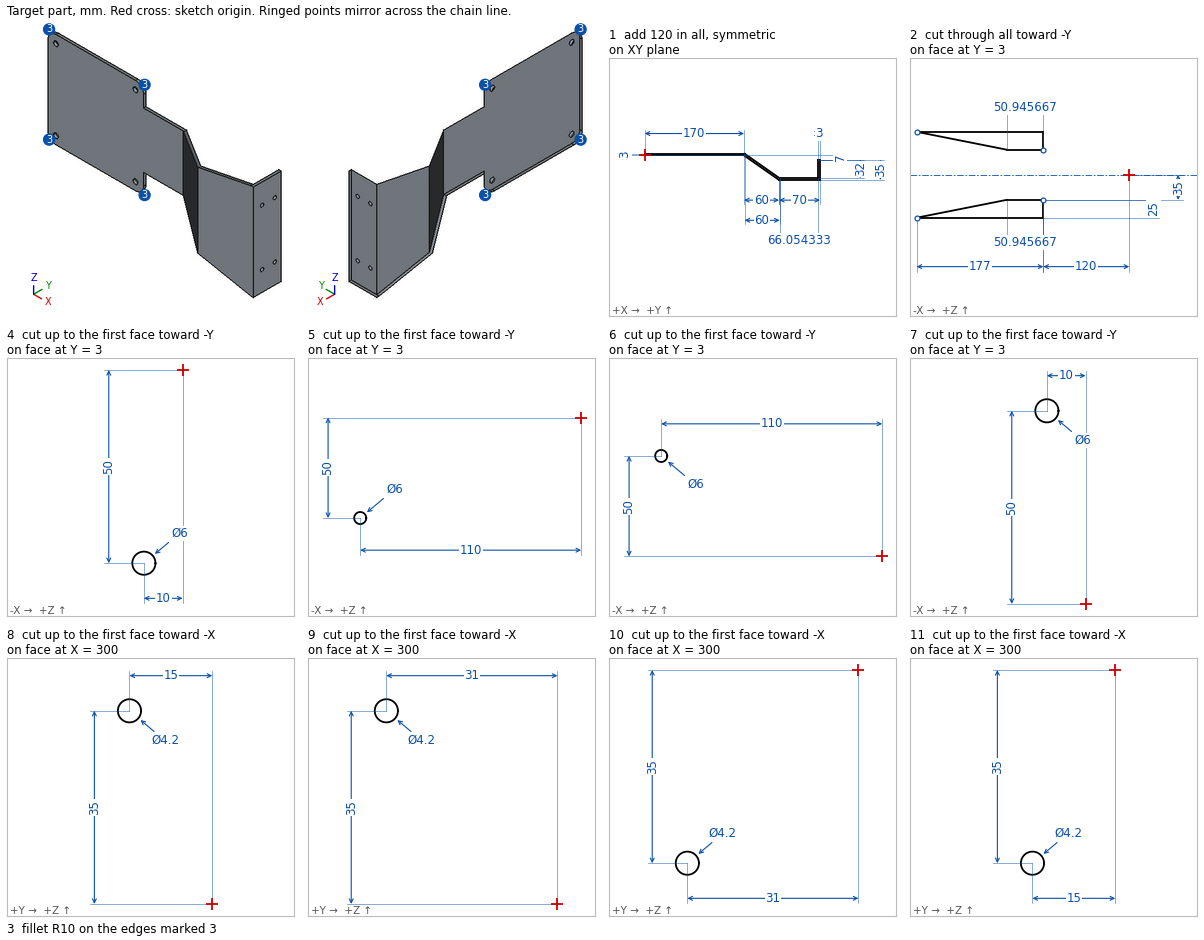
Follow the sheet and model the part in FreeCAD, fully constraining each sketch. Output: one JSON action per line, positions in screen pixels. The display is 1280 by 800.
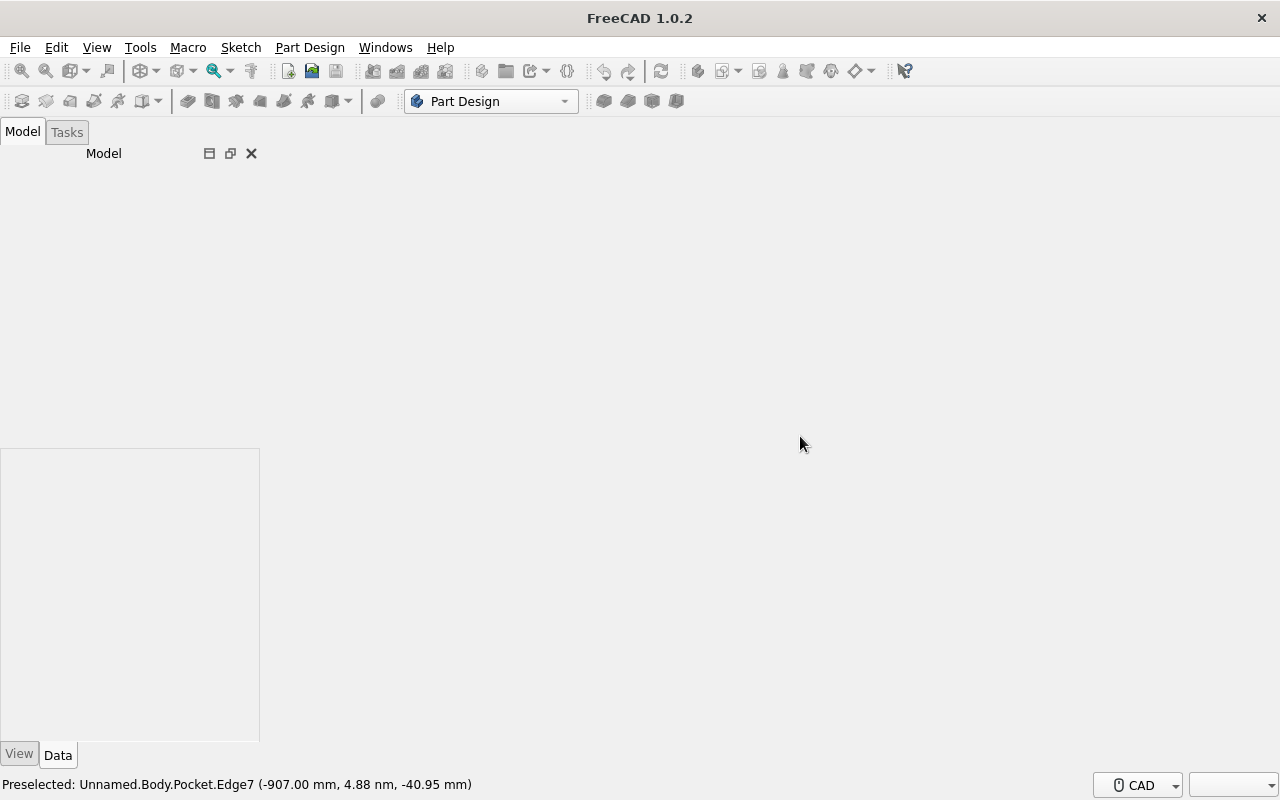
{"action": "left_click", "coordinate": [288, 72]}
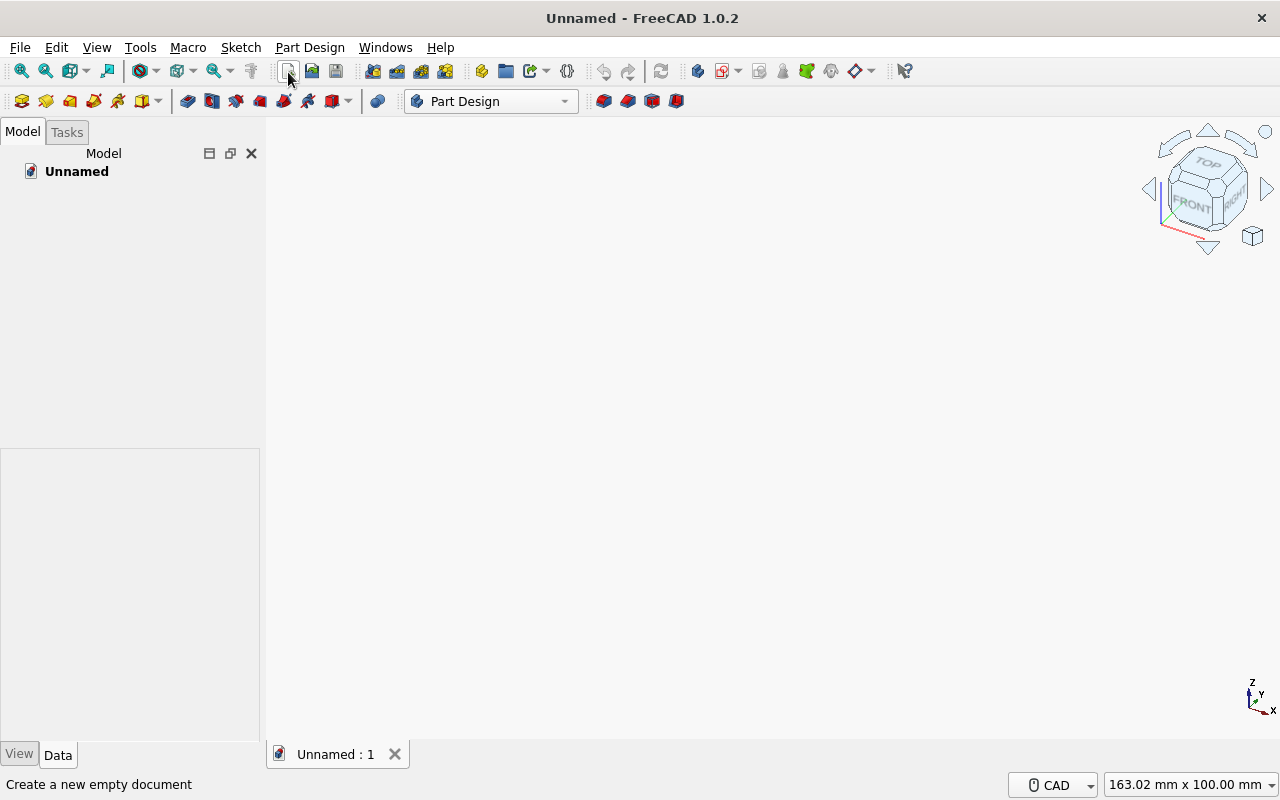
{"action": "left_click", "coordinate": [722, 72]}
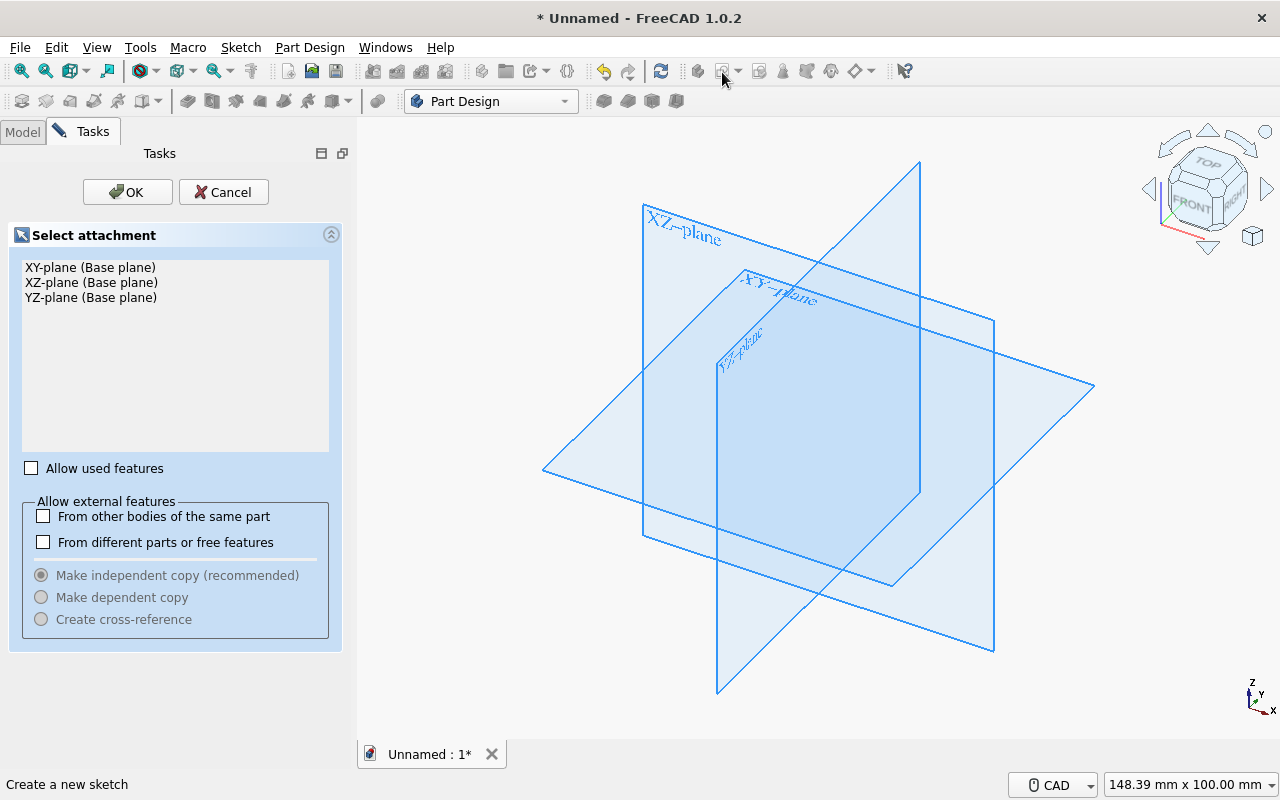
{"action": "left_click", "coordinate": [82, 268]}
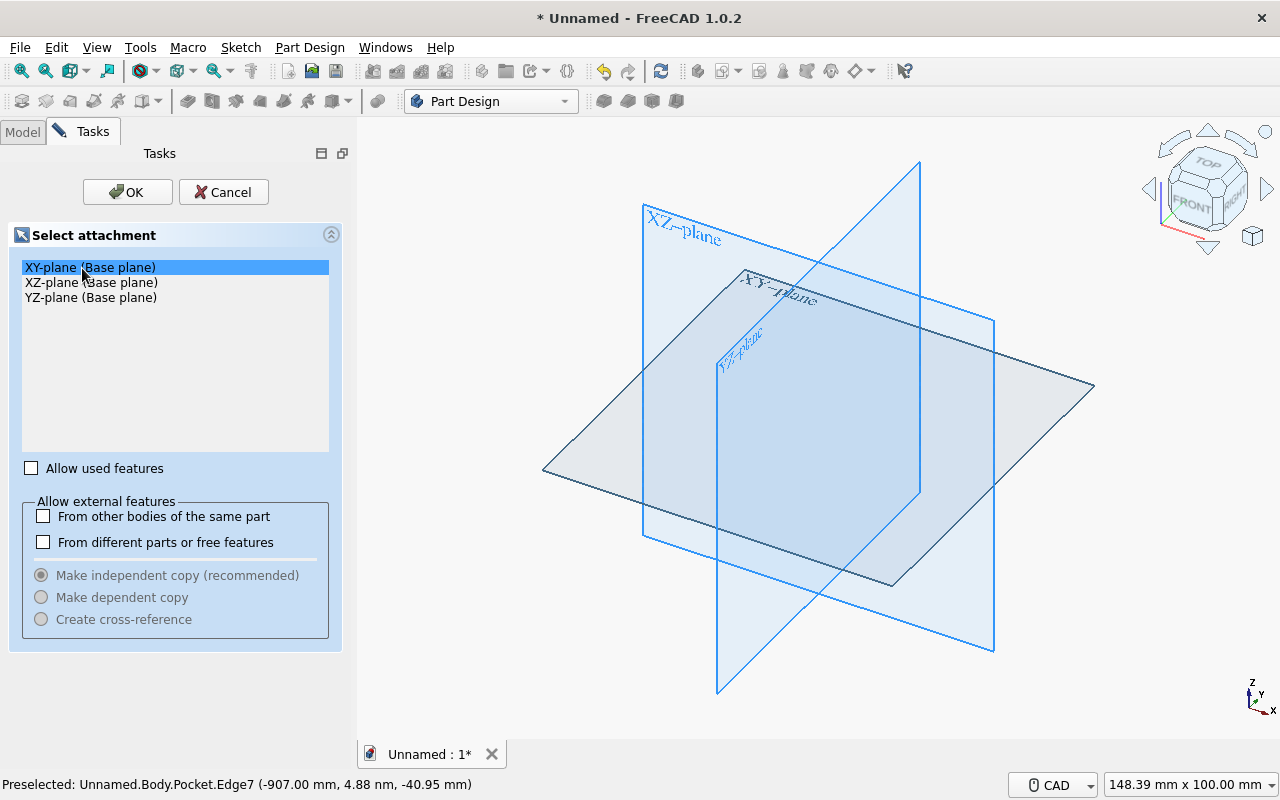
{"action": "left_click", "coordinate": [128, 192]}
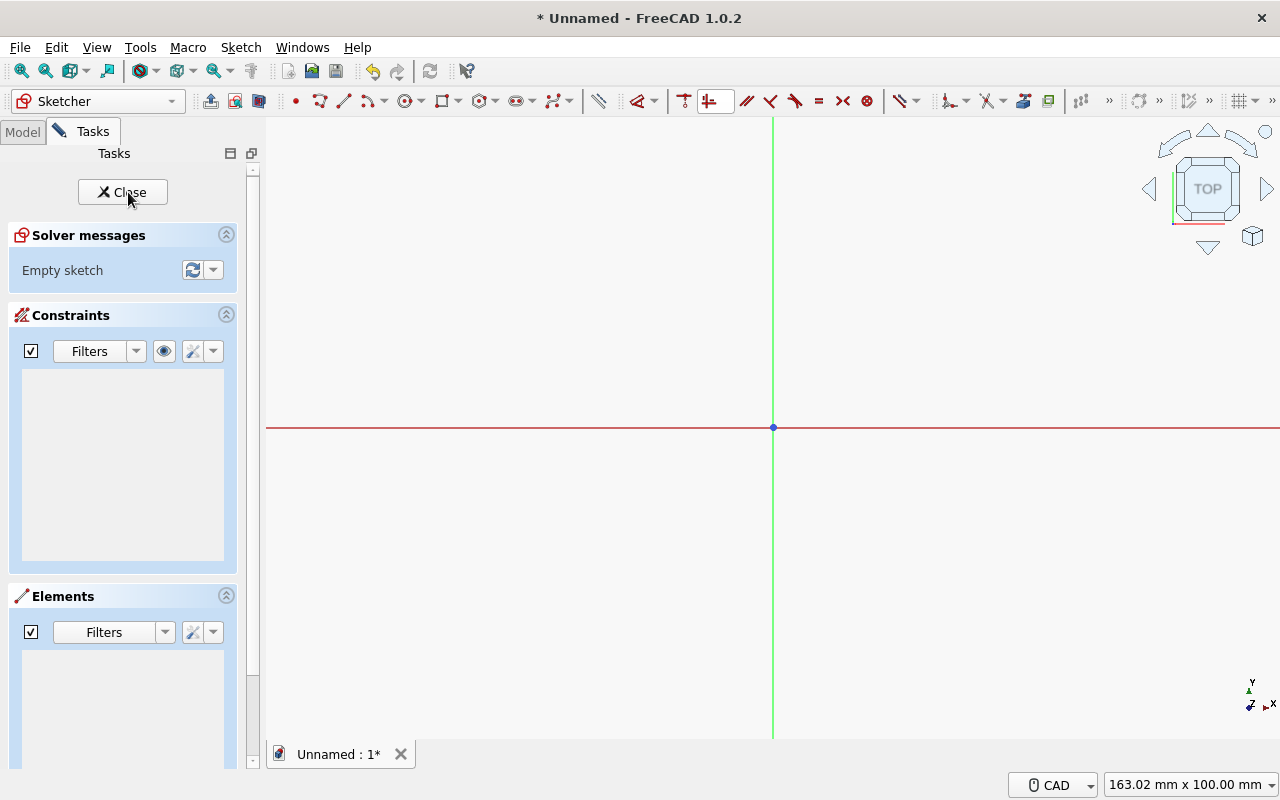
{"action": "scroll", "coordinate": [294, 376], "scroll_direction": "down", "scroll_amount": 6}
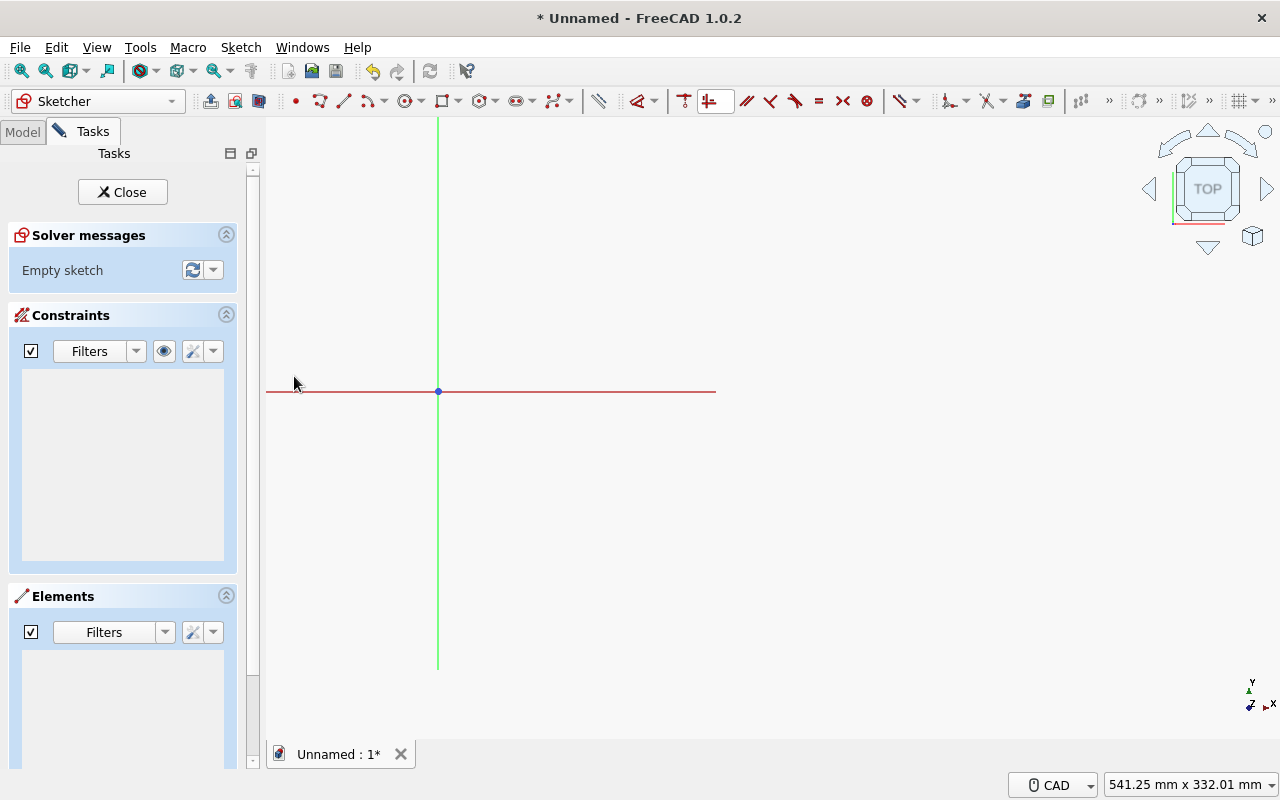
{"action": "left_click", "coordinate": [320, 102]}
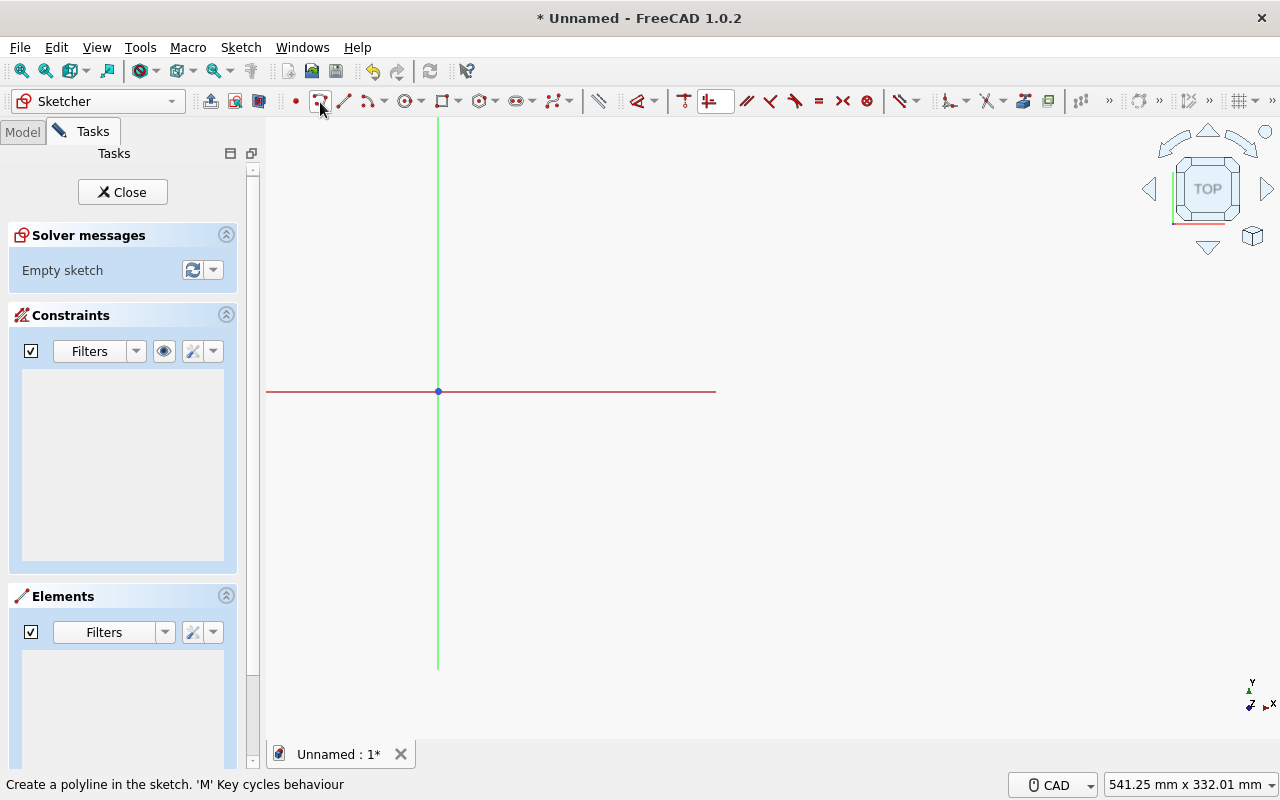
{"action": "left_click", "coordinate": [438, 392]}
{"action": "left_click", "coordinate": [757, 401]}
{"action": "left_click", "coordinate": [869, 471]}
{"action": "left_click", "coordinate": [1000, 471]}
{"action": "left_click", "coordinate": [1000, 405]}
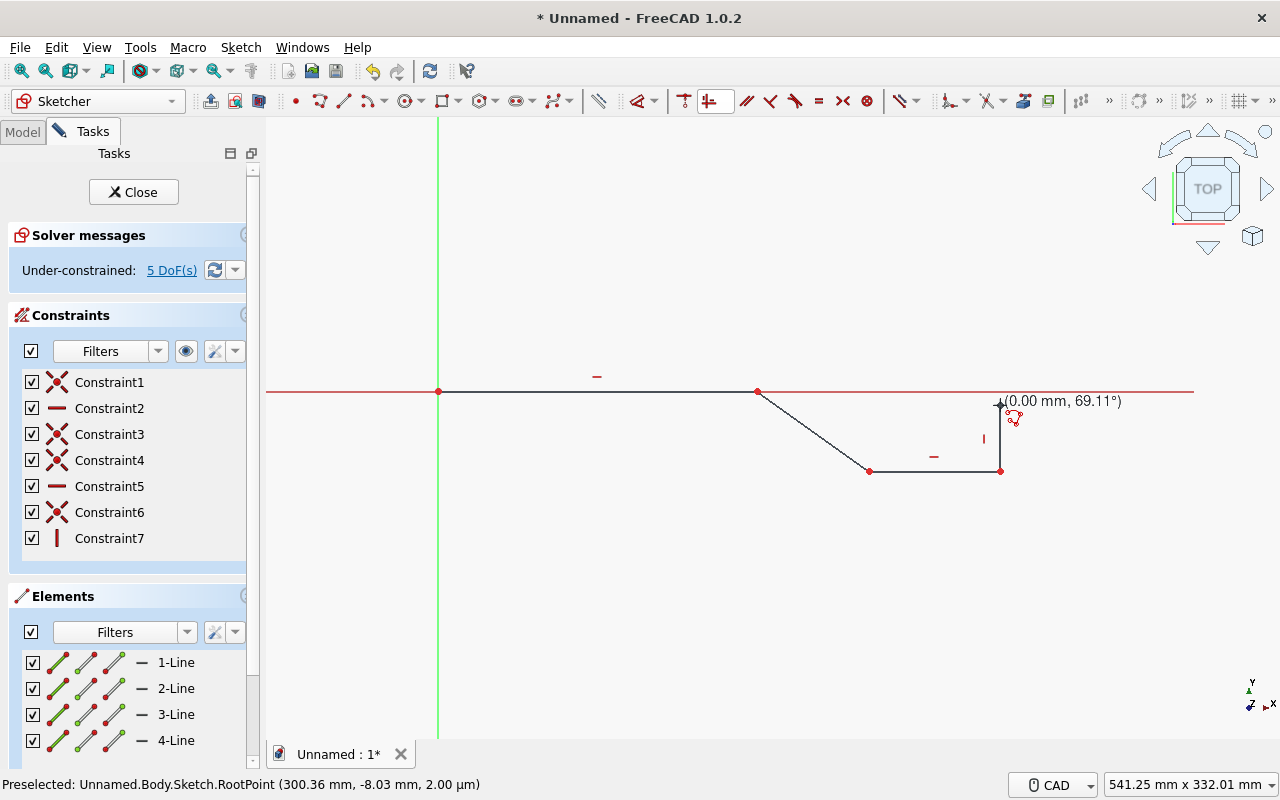
{"action": "scroll", "coordinate": [995, 405], "scroll_direction": "up", "scroll_amount": 6}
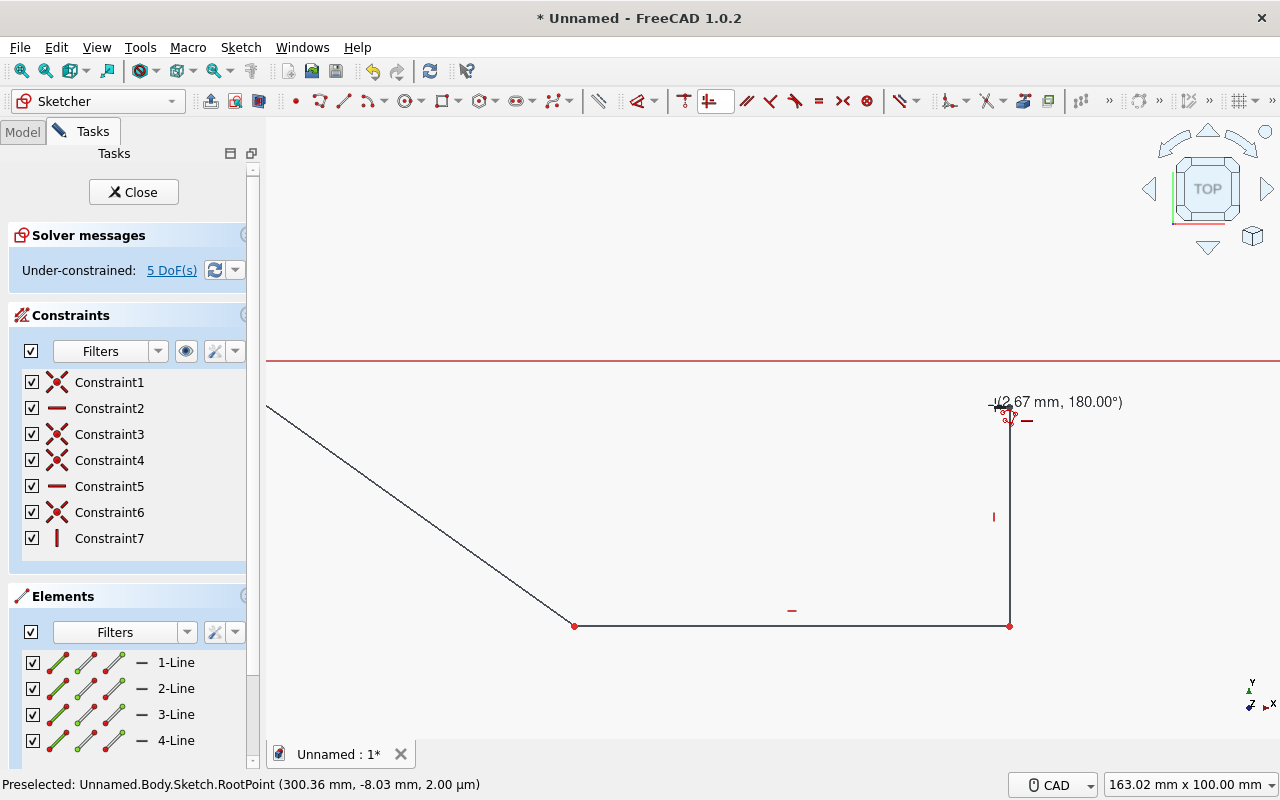
{"action": "left_click", "coordinate": [992, 404]}
{"action": "left_click", "coordinate": [992, 603]}
{"action": "left_click", "coordinate": [581, 603]}